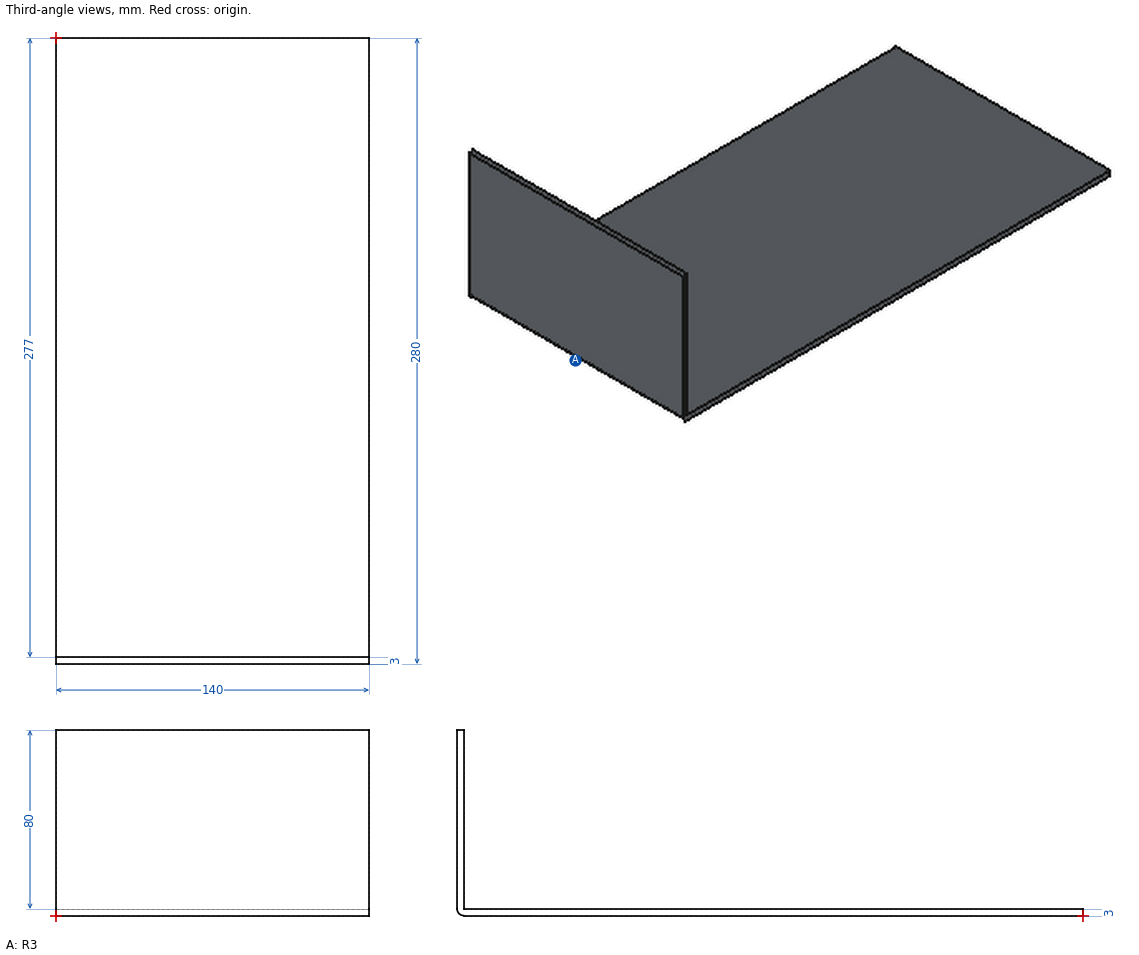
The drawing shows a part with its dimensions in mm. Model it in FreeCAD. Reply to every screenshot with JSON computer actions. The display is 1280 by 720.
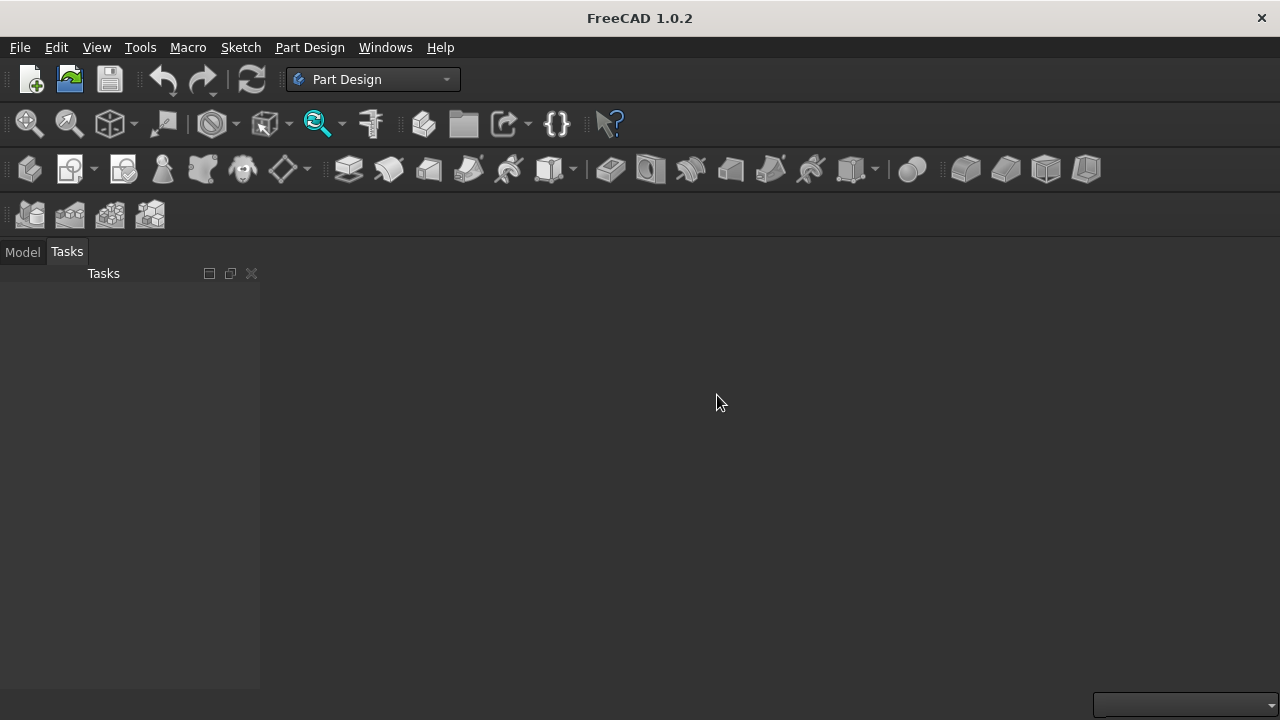
{"action": "left_click", "coordinate": [30, 80]}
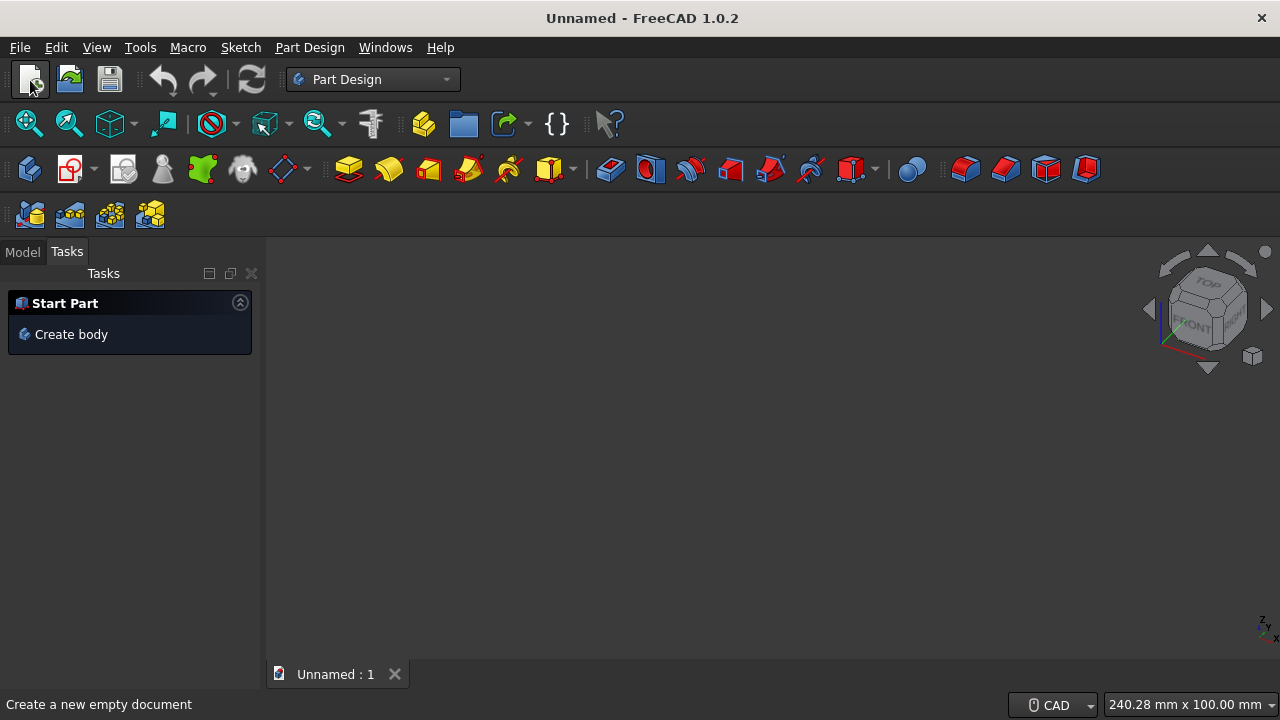
{"action": "left_click", "coordinate": [70, 170]}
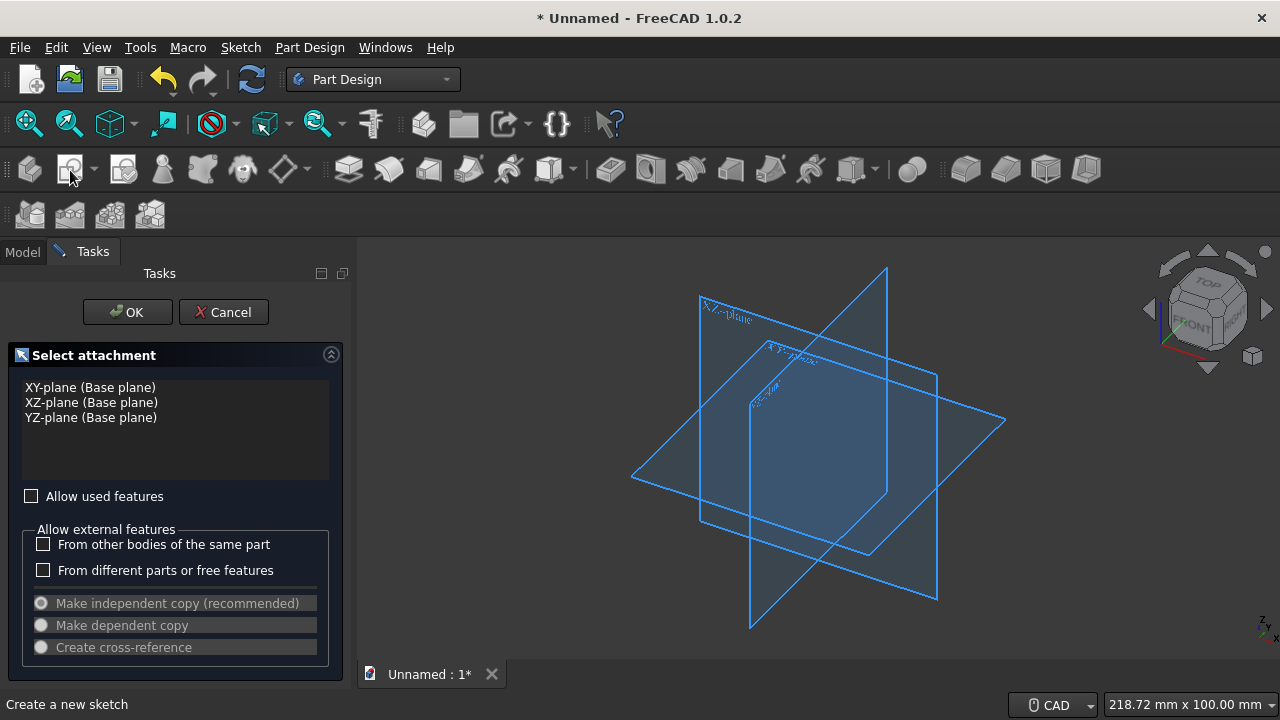
{"action": "left_click", "coordinate": [82, 388]}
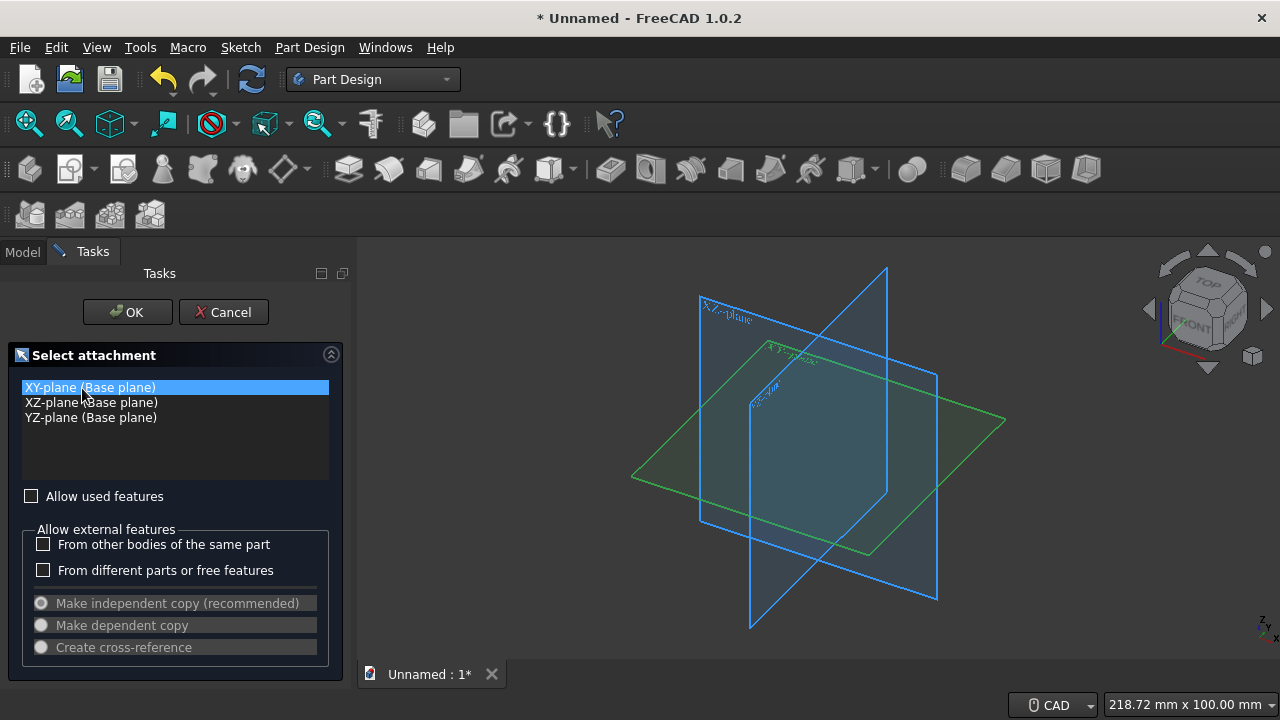
{"action": "left_click", "coordinate": [128, 312]}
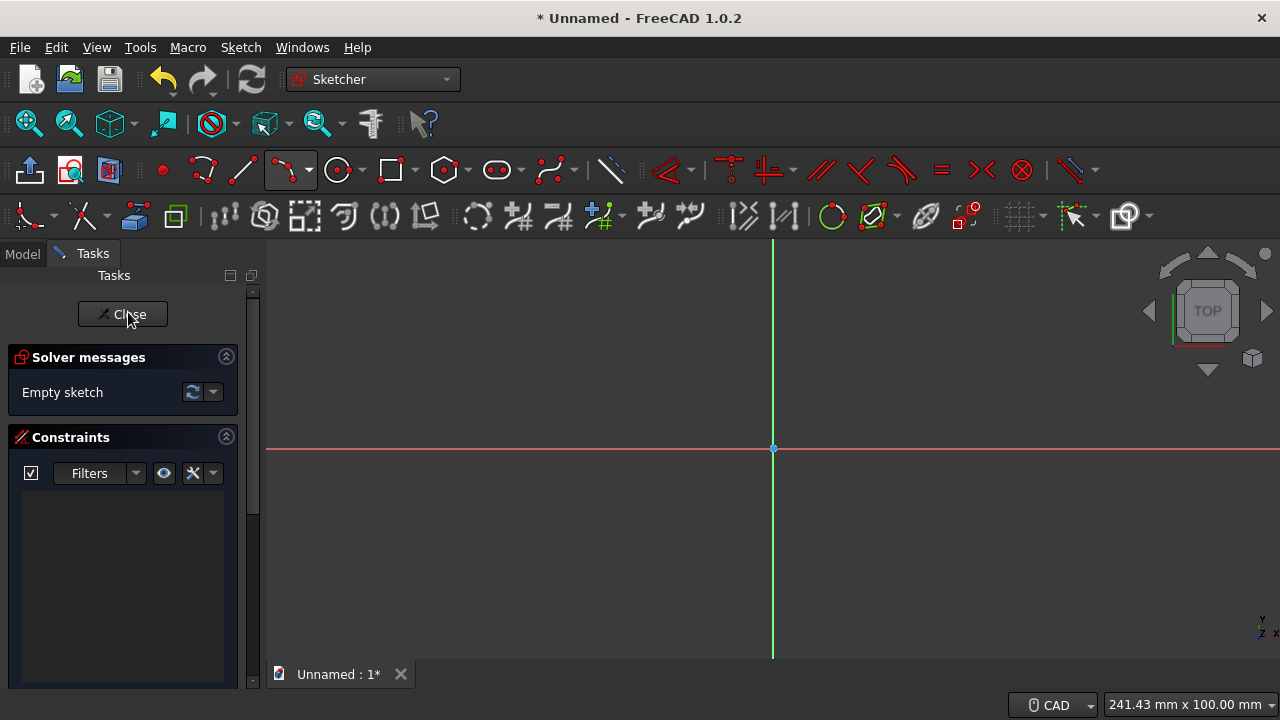
{"action": "scroll", "coordinate": [613, 300], "scroll_direction": "down", "scroll_amount": 8}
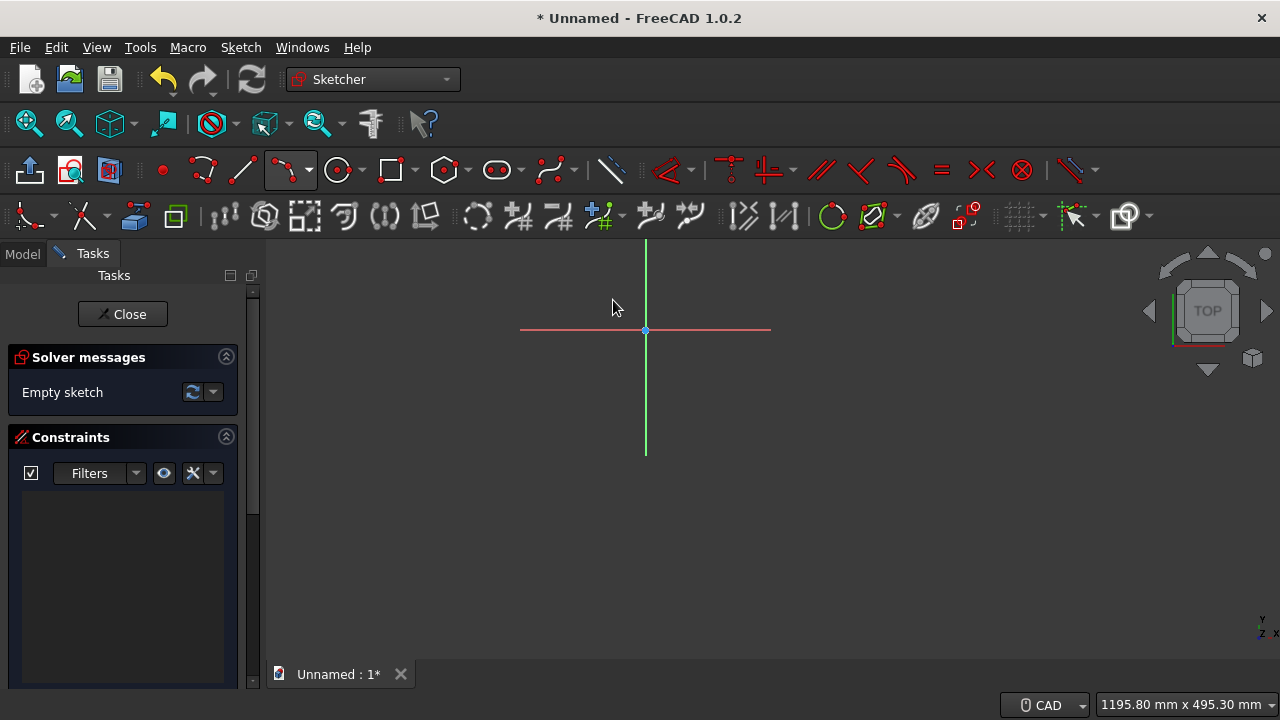
{"action": "left_click", "coordinate": [392, 170]}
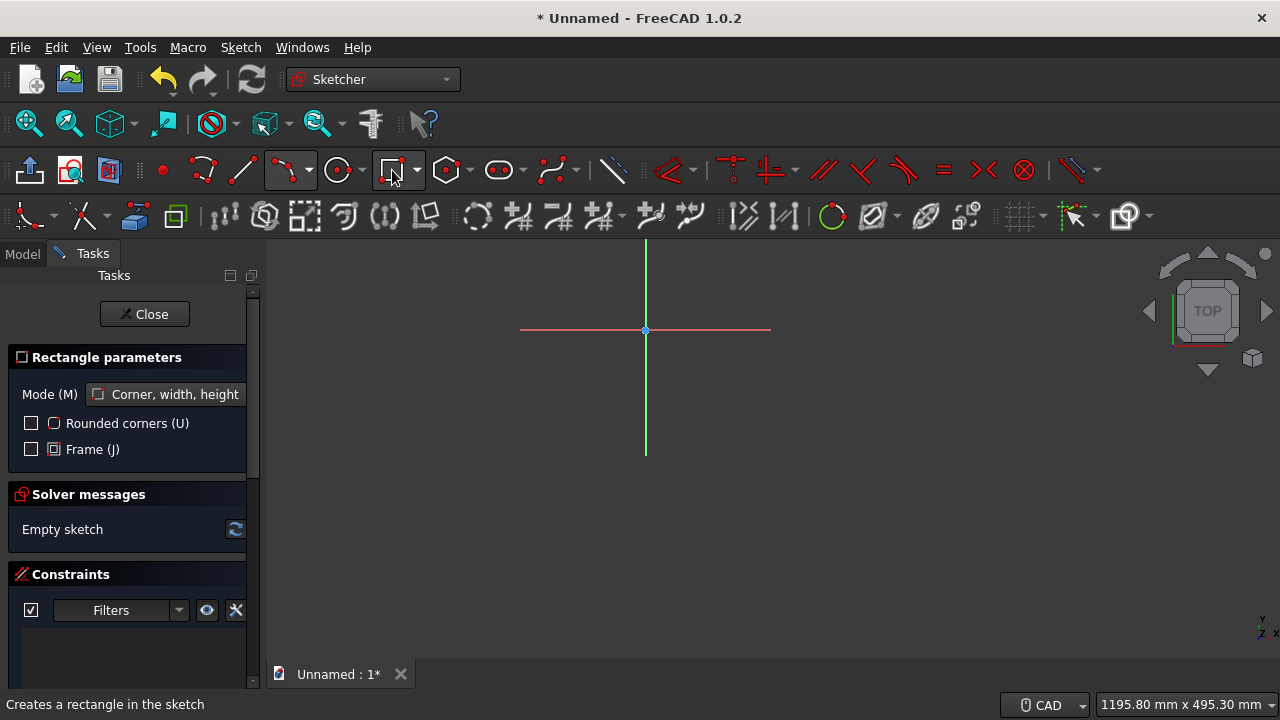
{"action": "left_click", "coordinate": [646, 330]}
{"action": "mouse_move", "coordinate": [764, 568]}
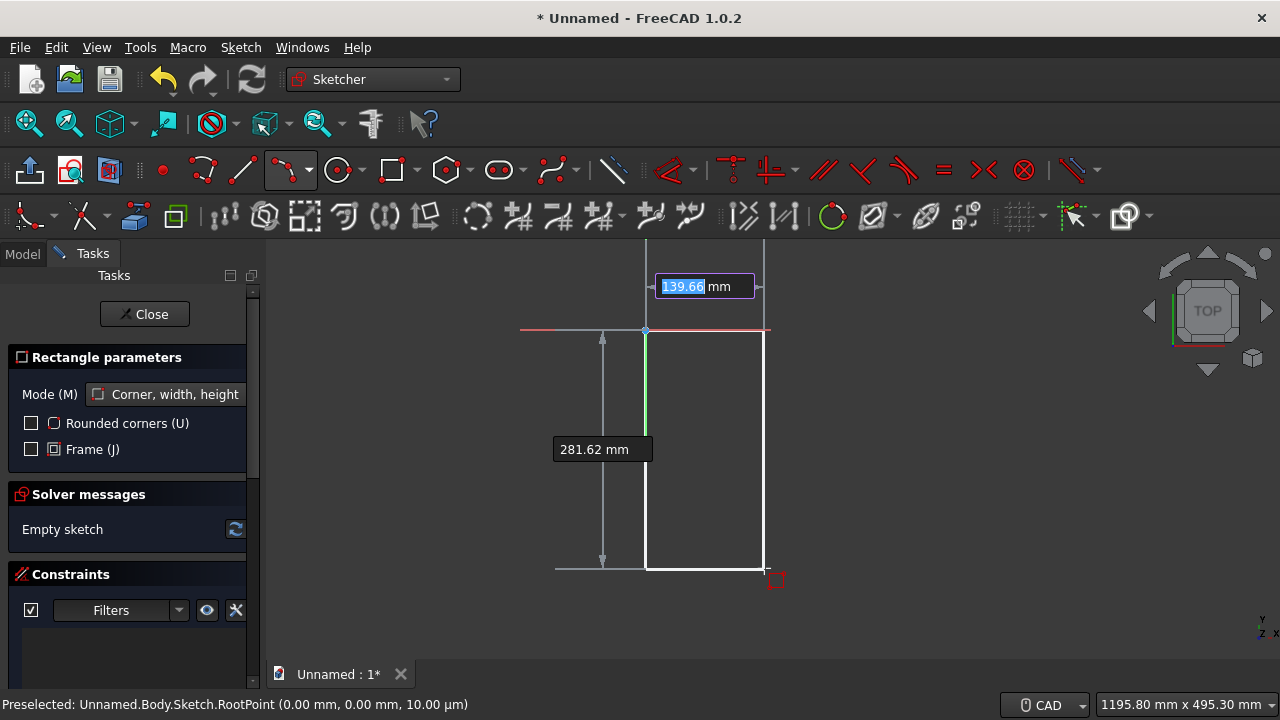
{"action": "type", "text": "140"}
{"action": "key", "text": "Tab"}
{"action": "type", "text": "280"}
{"action": "key", "text": "Return"}
{"action": "key", "text": "Escape"}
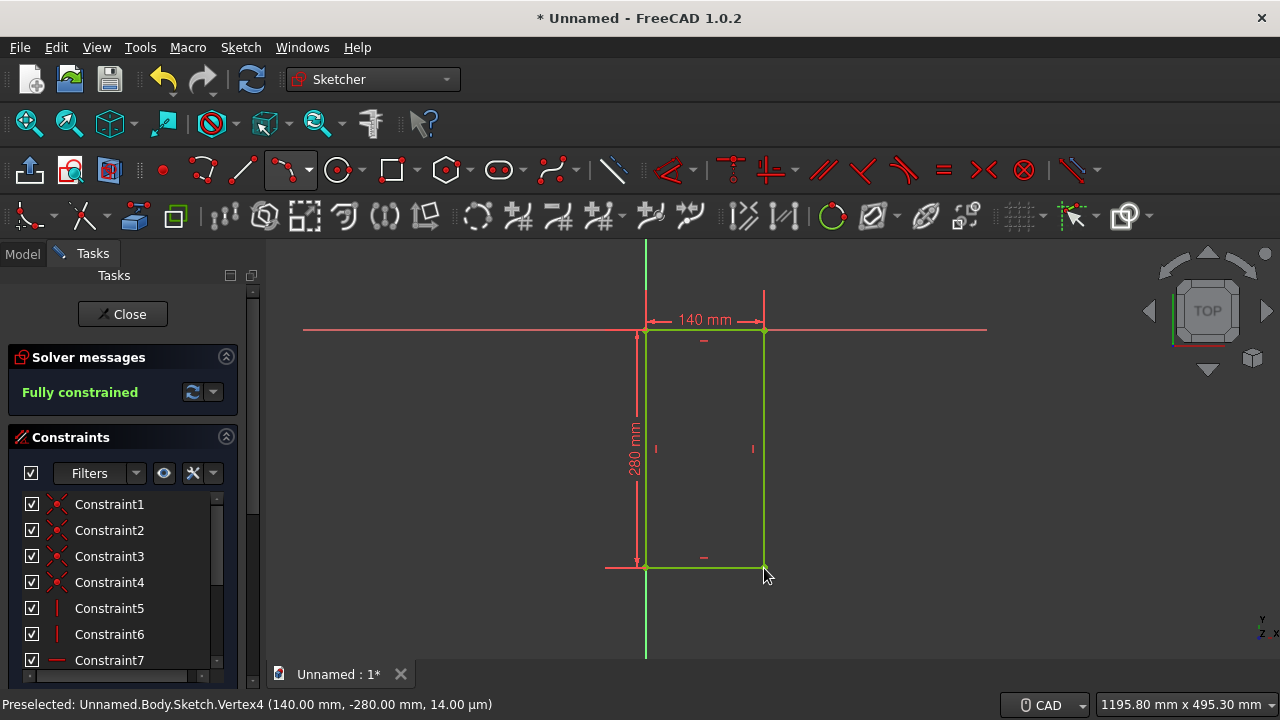
{"action": "left_click", "coordinate": [123, 314]}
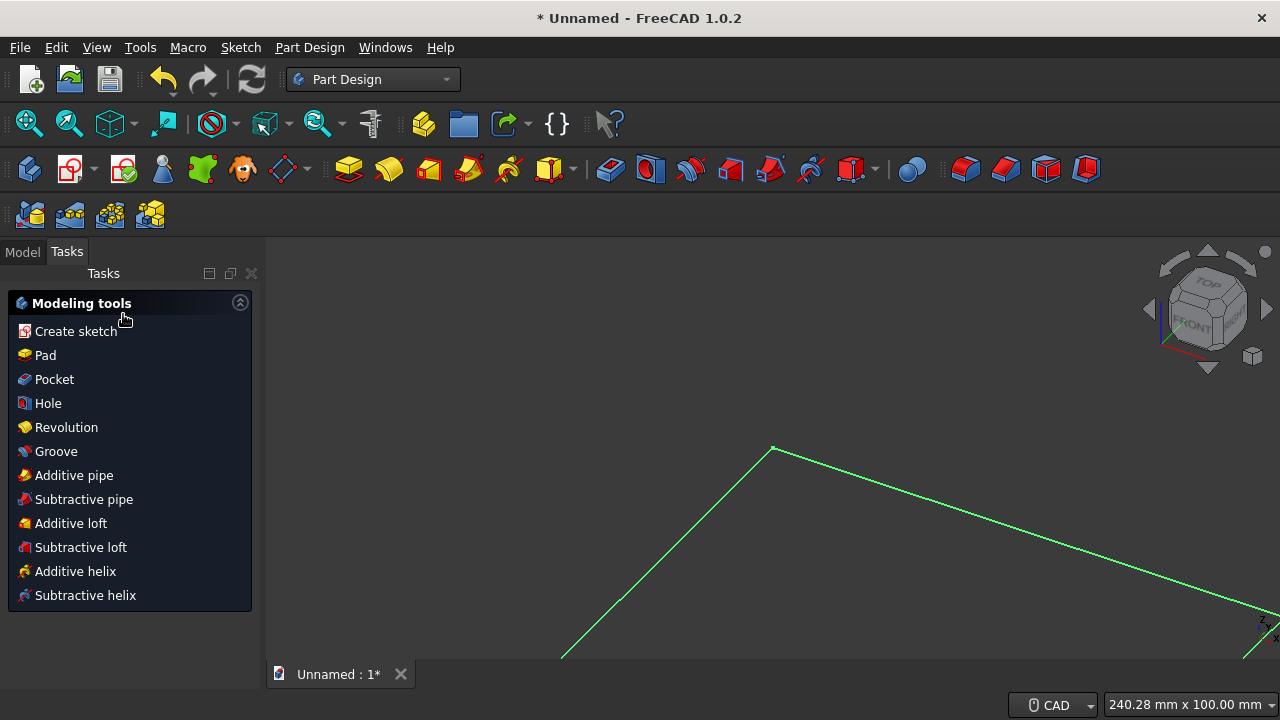
{"action": "left_click", "coordinate": [350, 170]}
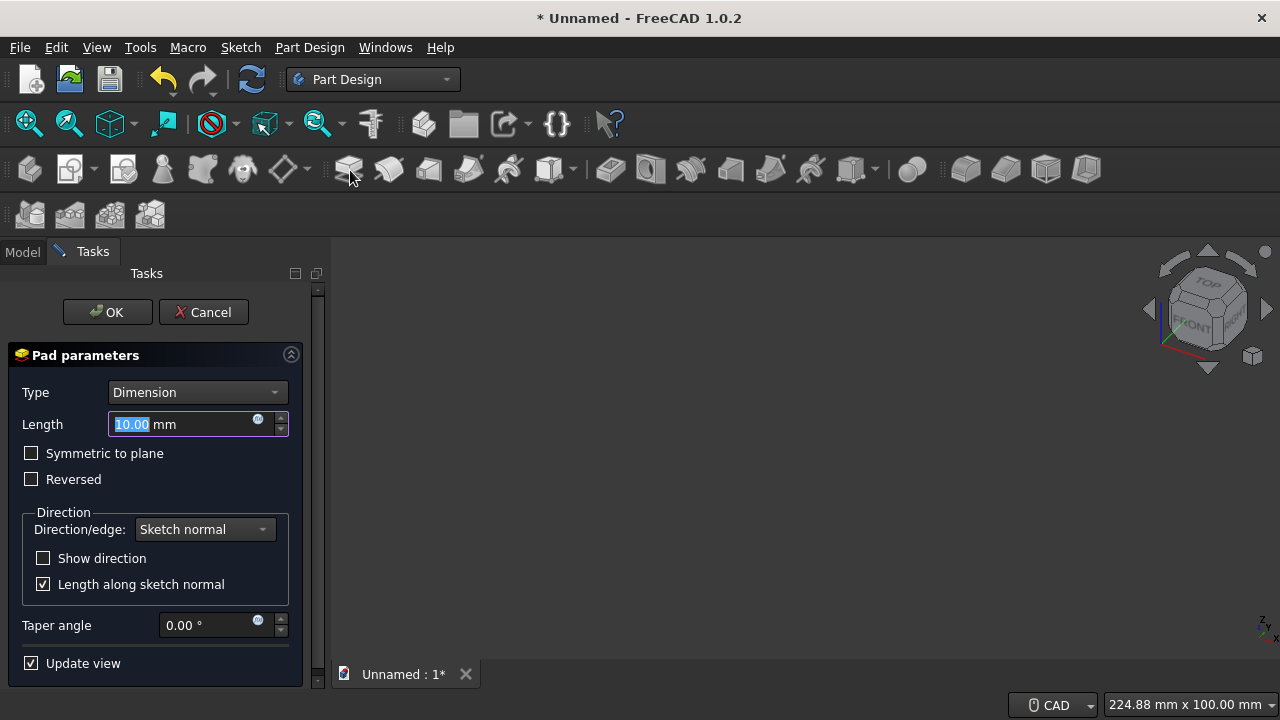
{"action": "type", "text": "3"}
{"action": "key", "text": "Tab"}